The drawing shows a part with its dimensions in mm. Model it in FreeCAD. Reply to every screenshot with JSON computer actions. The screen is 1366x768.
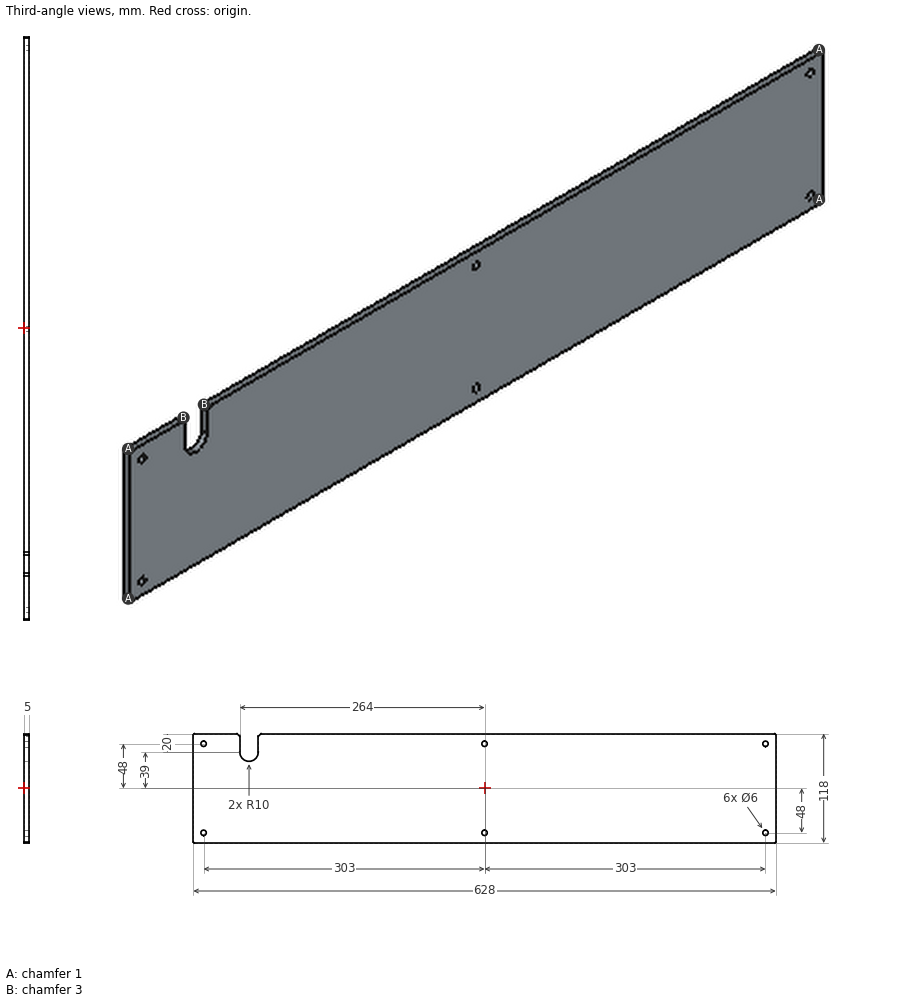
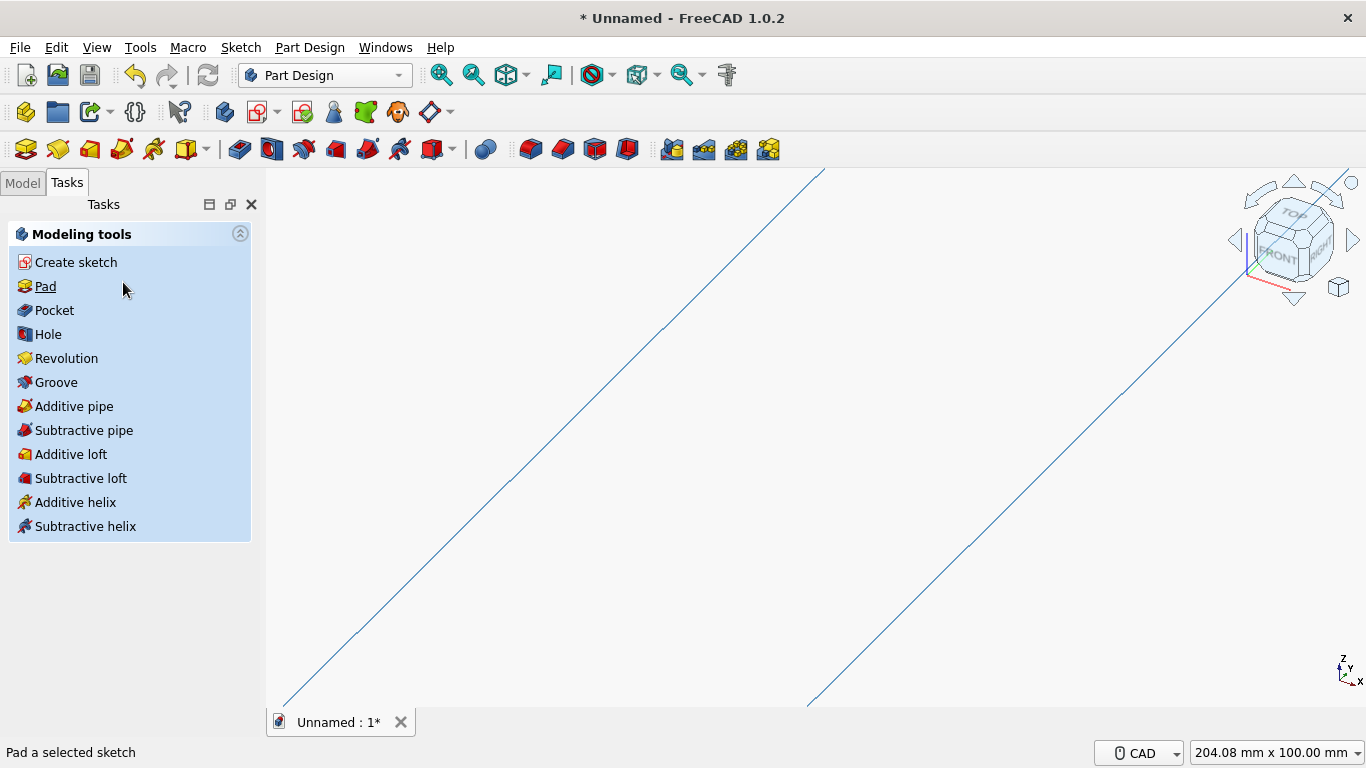
{"action": "left_click", "coordinate": [26, 150]}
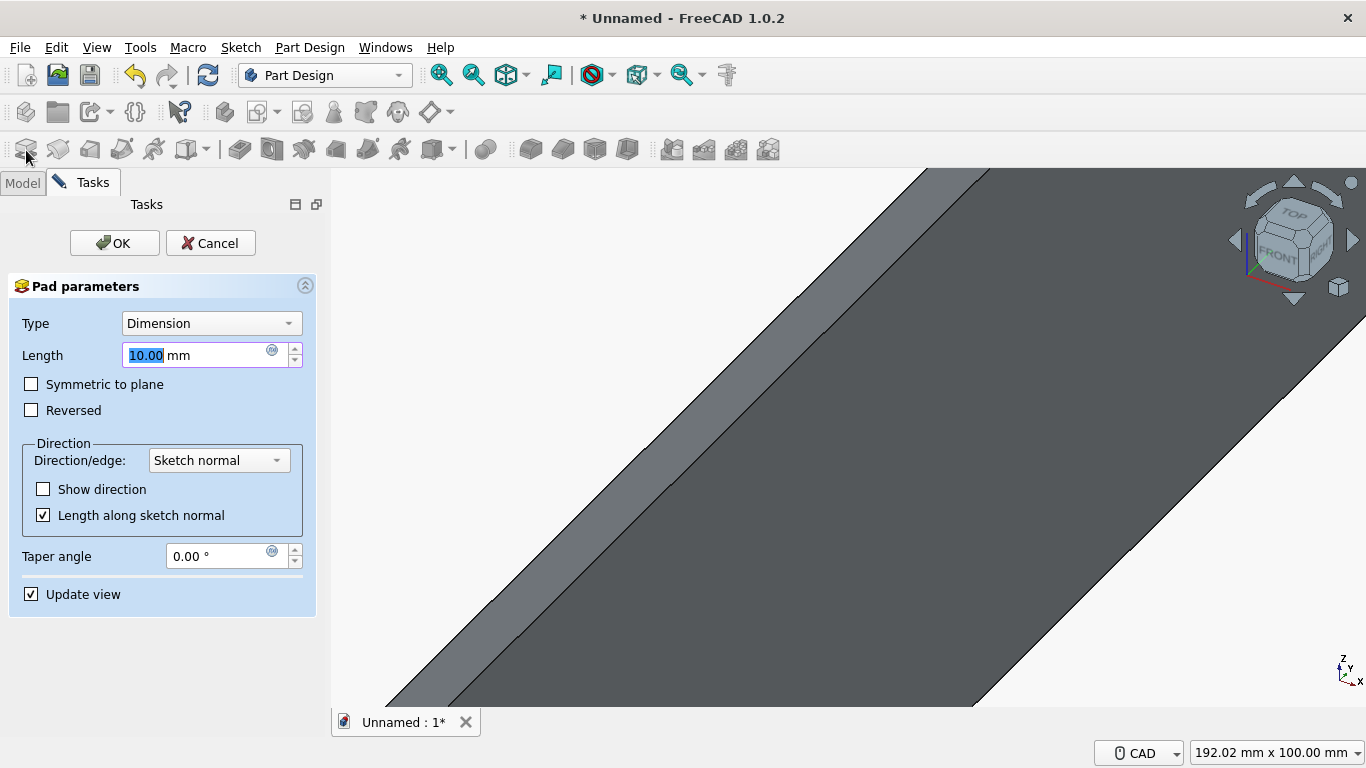
{"action": "type", "text": "5"}
{"action": "key", "text": "Tab"}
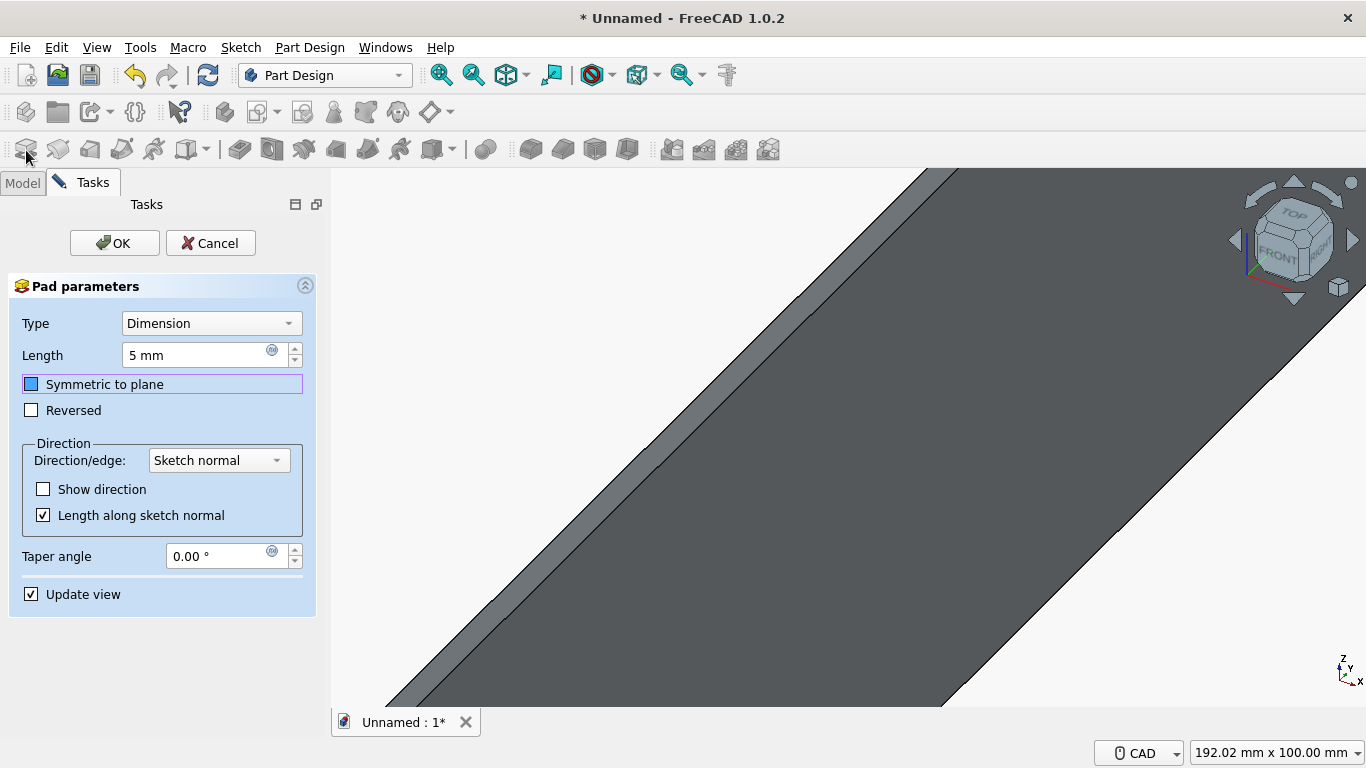
{"action": "left_click", "coordinate": [115, 243]}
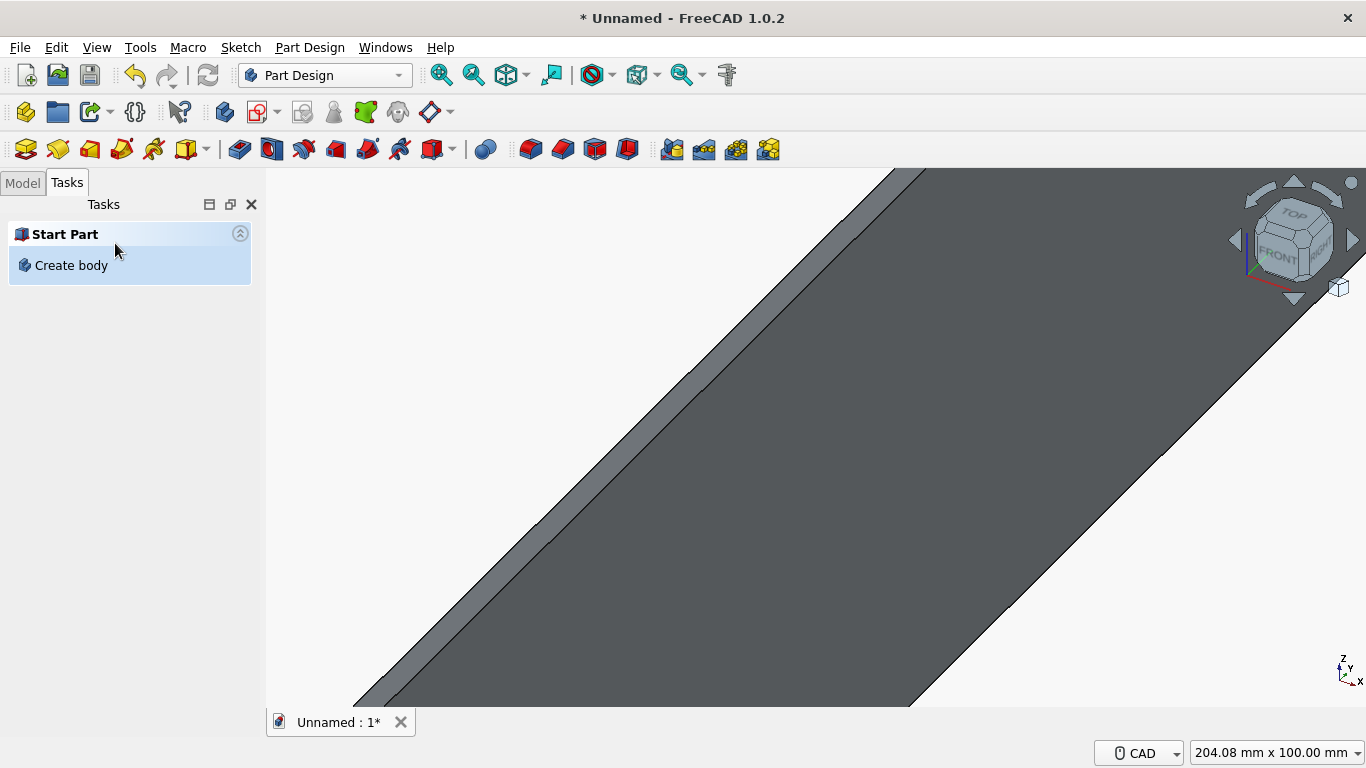
{"action": "left_click", "coordinate": [442, 76]}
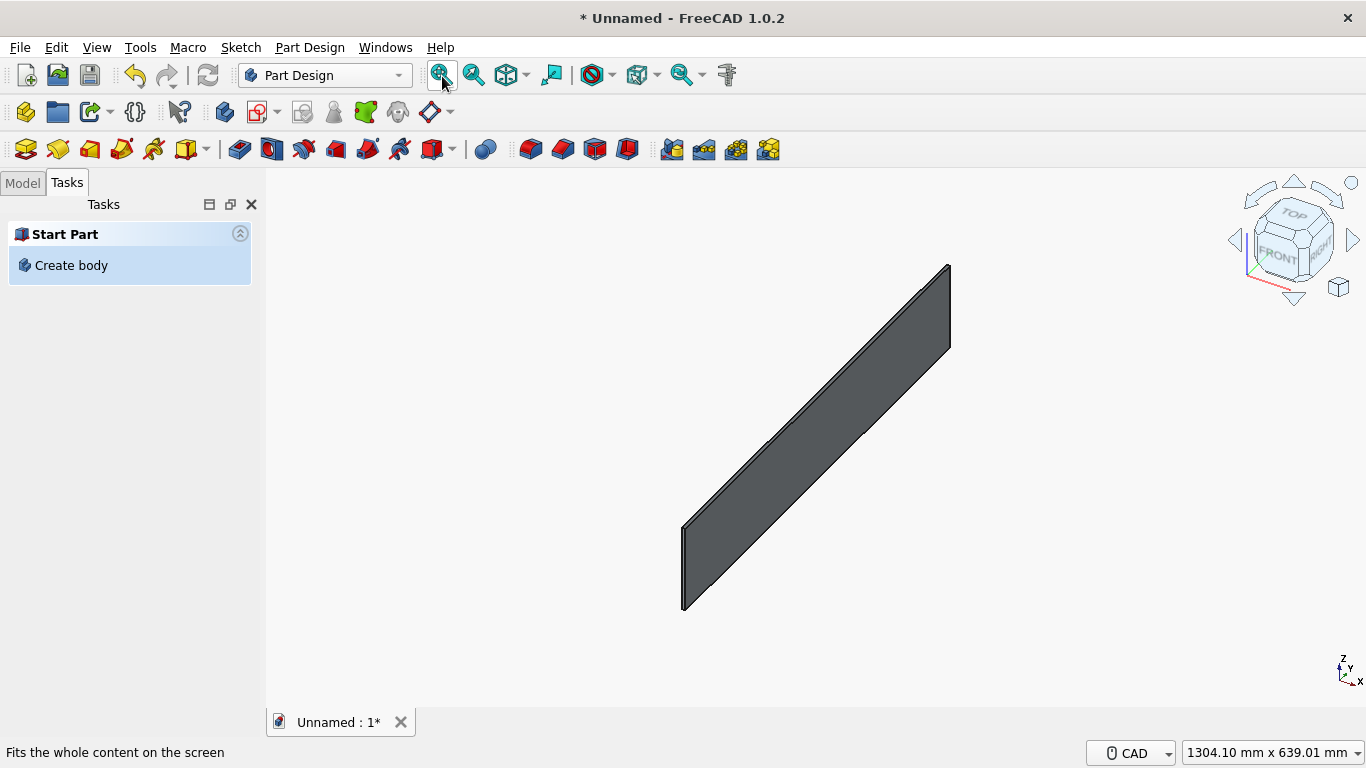
{"action": "scroll", "coordinate": [948, 264], "scroll_direction": "up", "scroll_amount": 12}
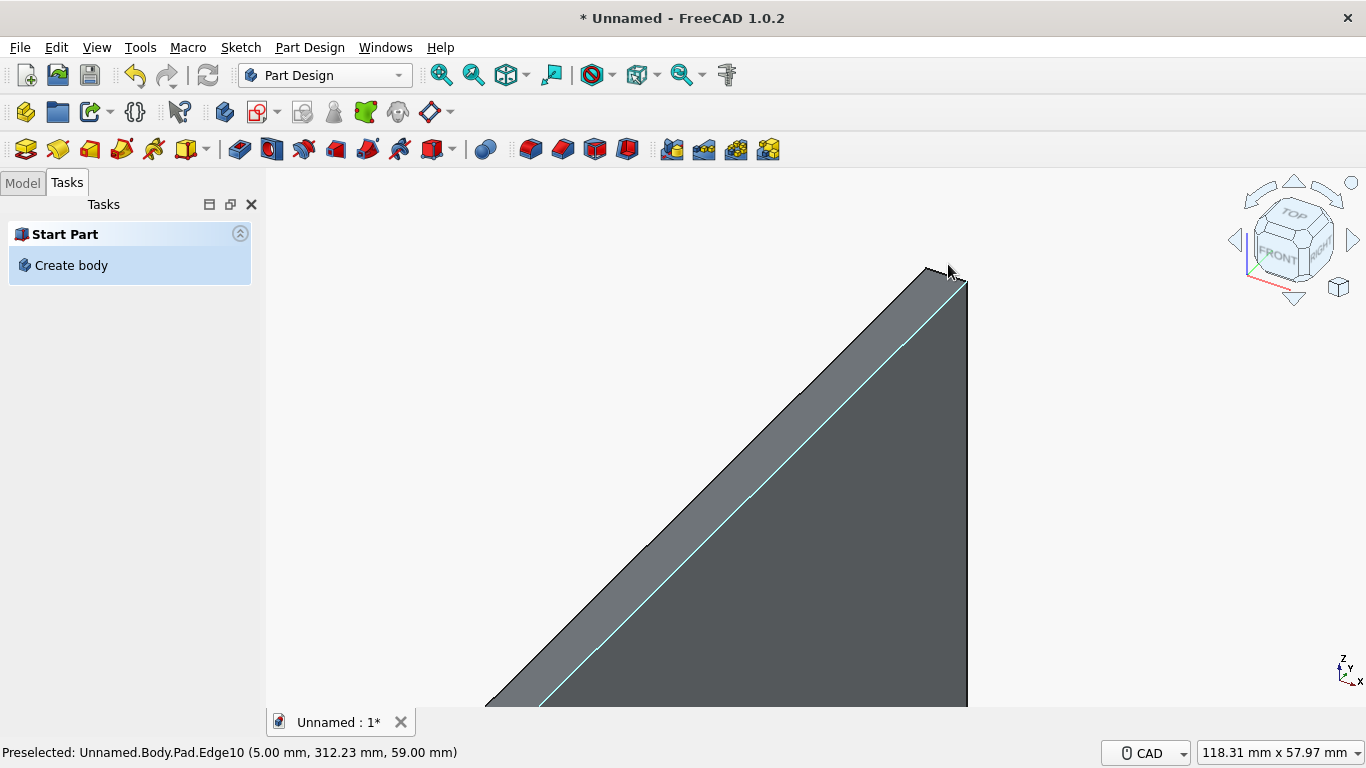
{"action": "left_click", "coordinate": [442, 76]}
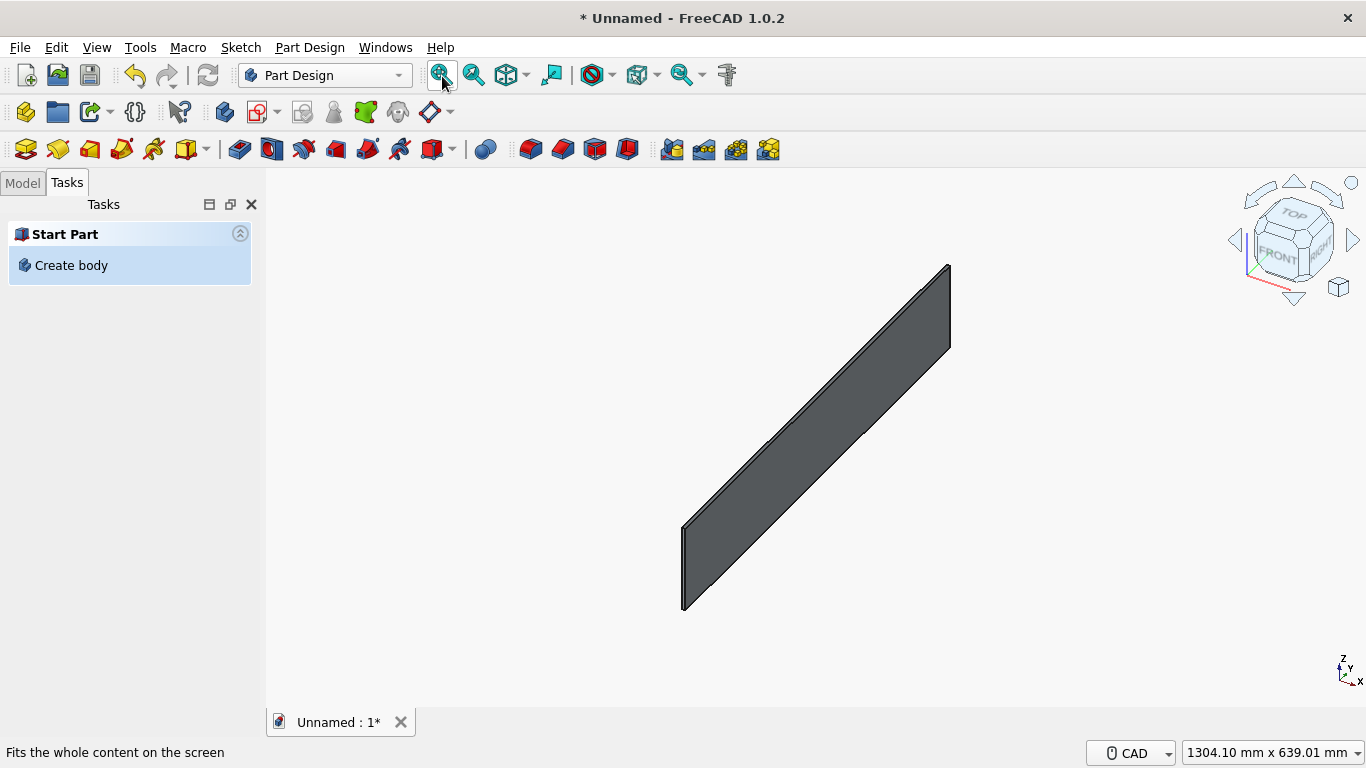
{"action": "key", "text": "0"}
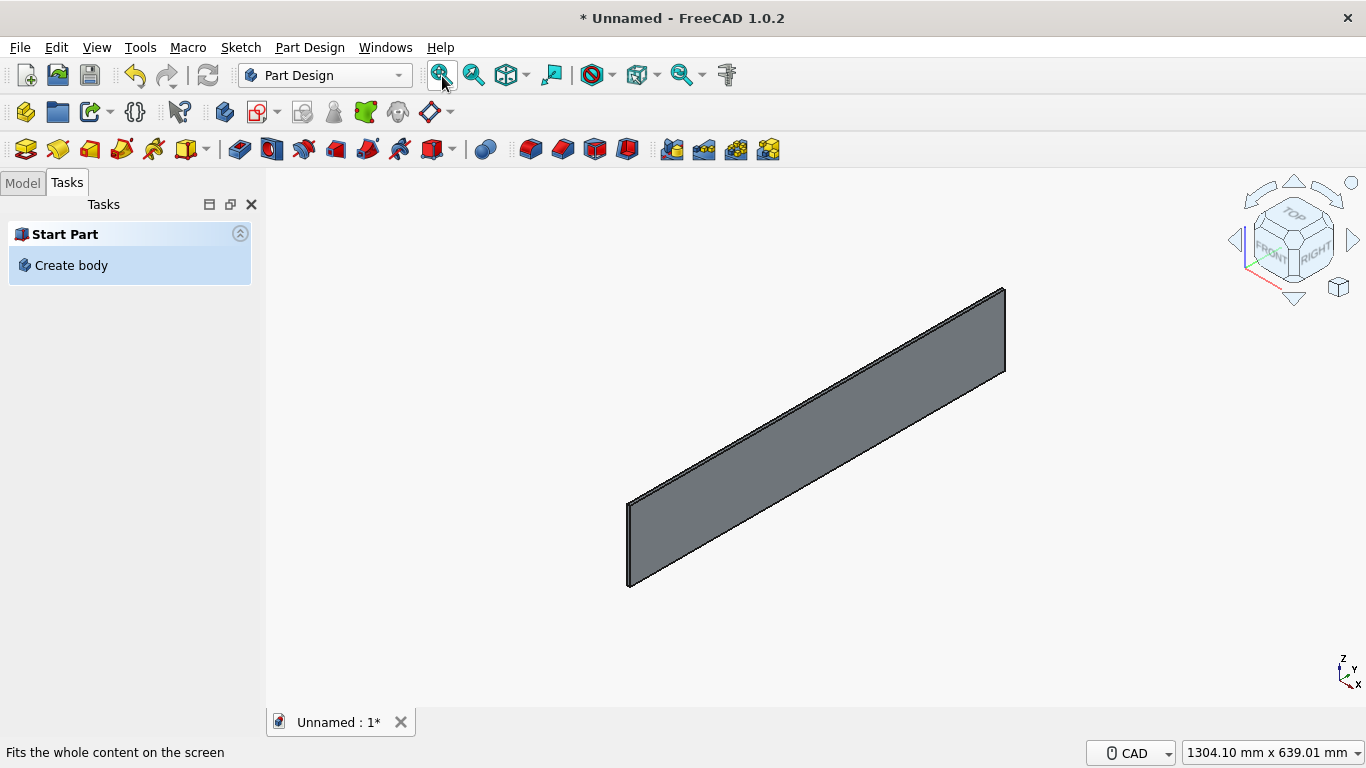
{"action": "scroll", "coordinate": [1003, 288], "scroll_direction": "up", "scroll_amount": 12}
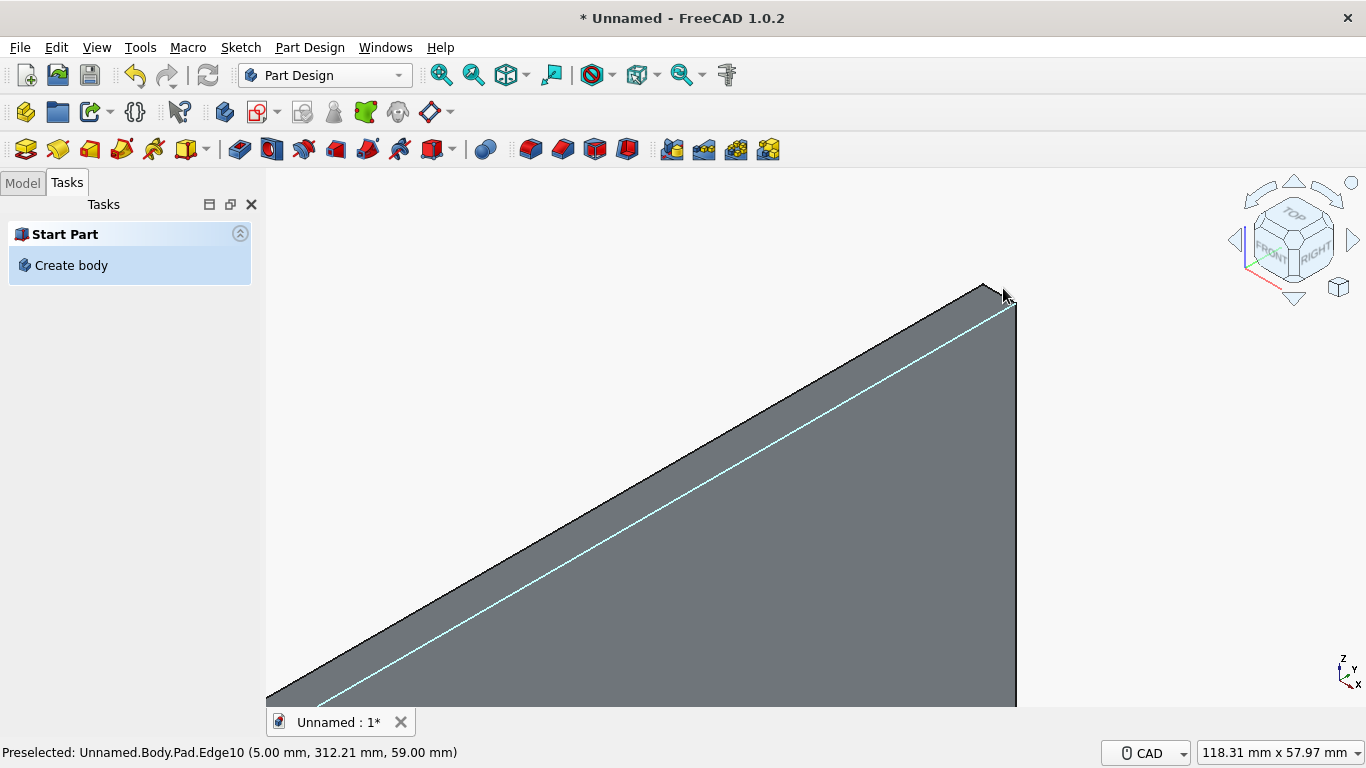
{"action": "left_click", "coordinate": [442, 76]}